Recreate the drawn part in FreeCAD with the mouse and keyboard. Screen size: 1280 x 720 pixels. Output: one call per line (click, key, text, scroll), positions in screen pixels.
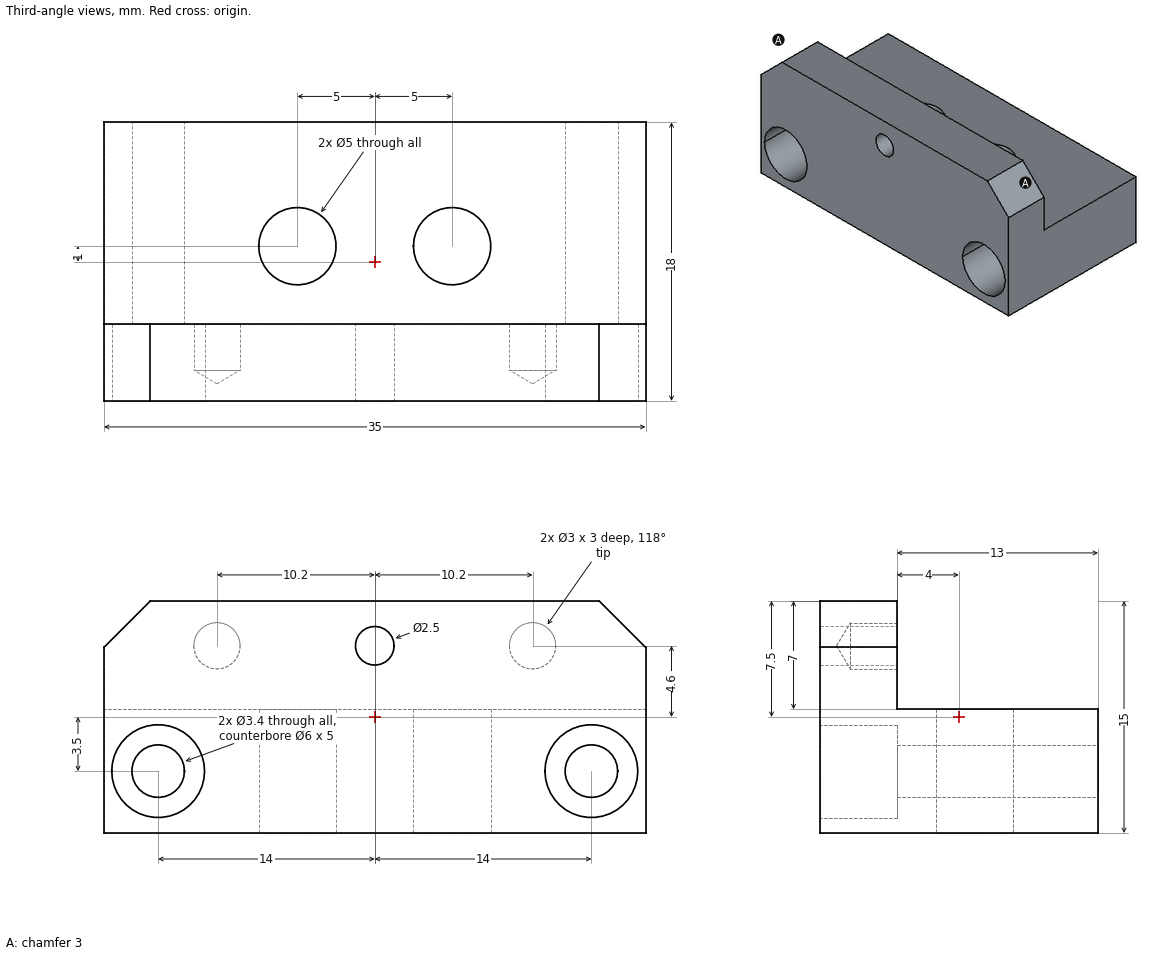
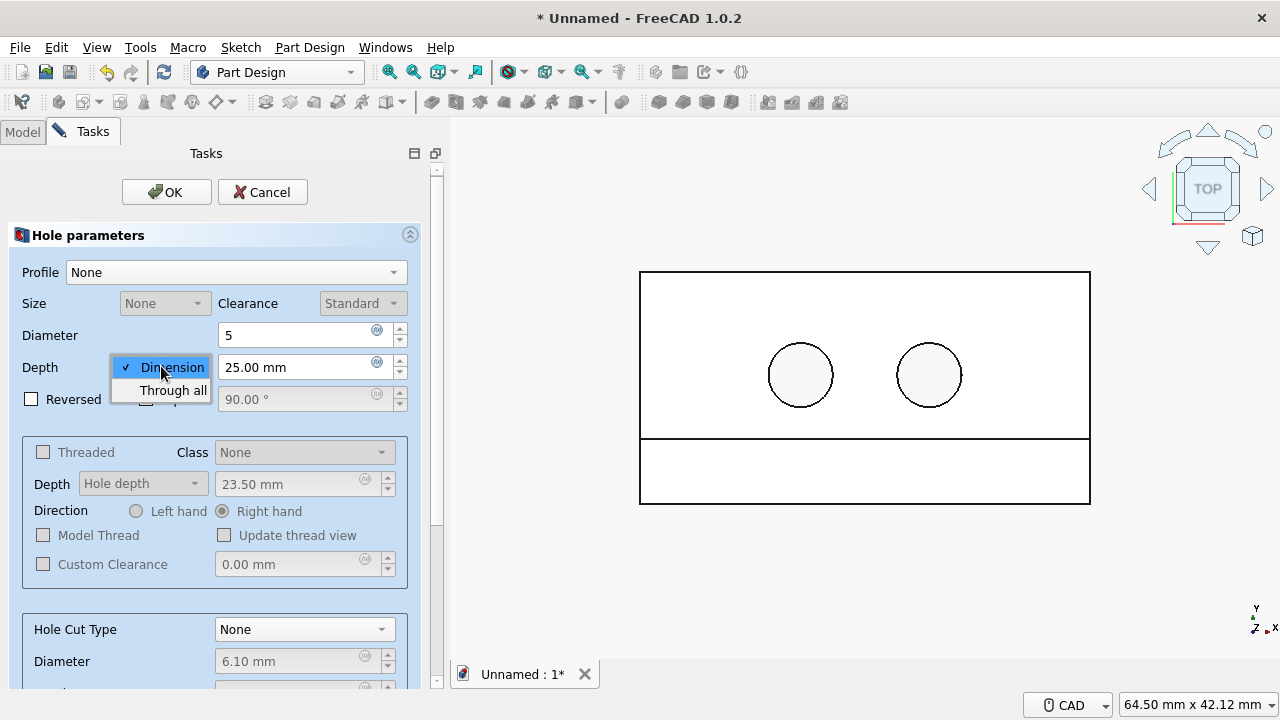
click(160, 390)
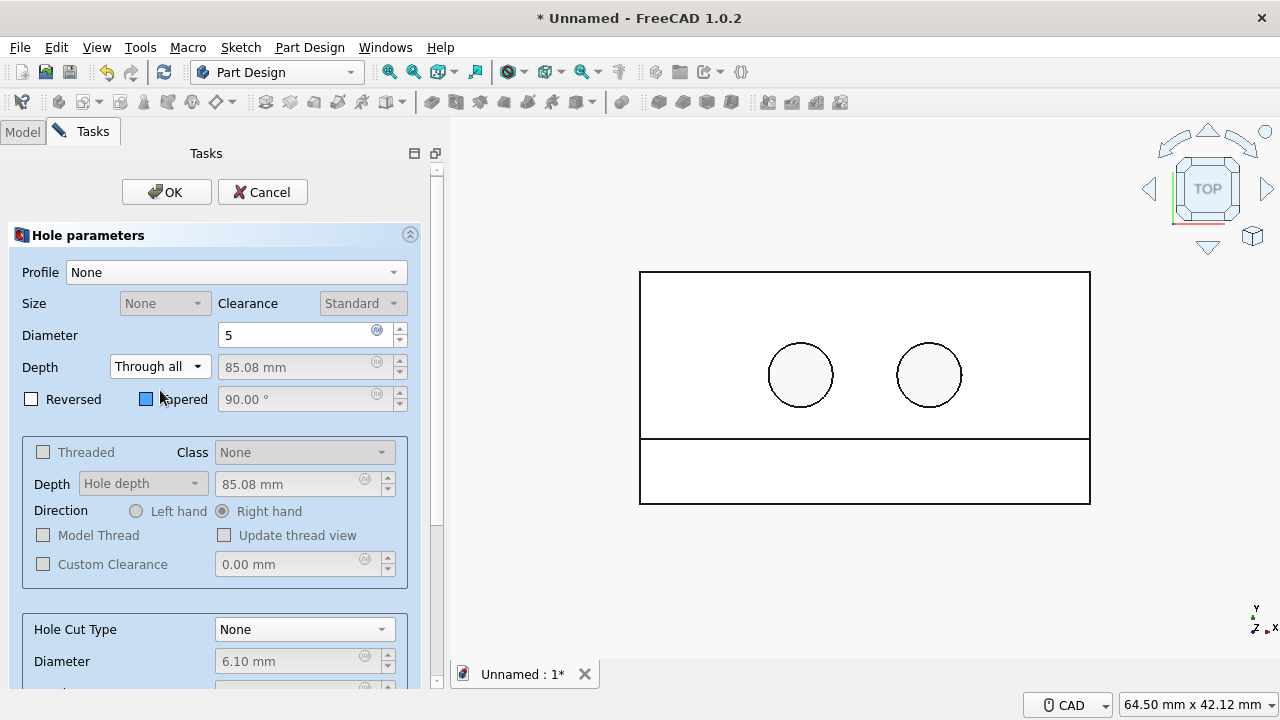
click(167, 192)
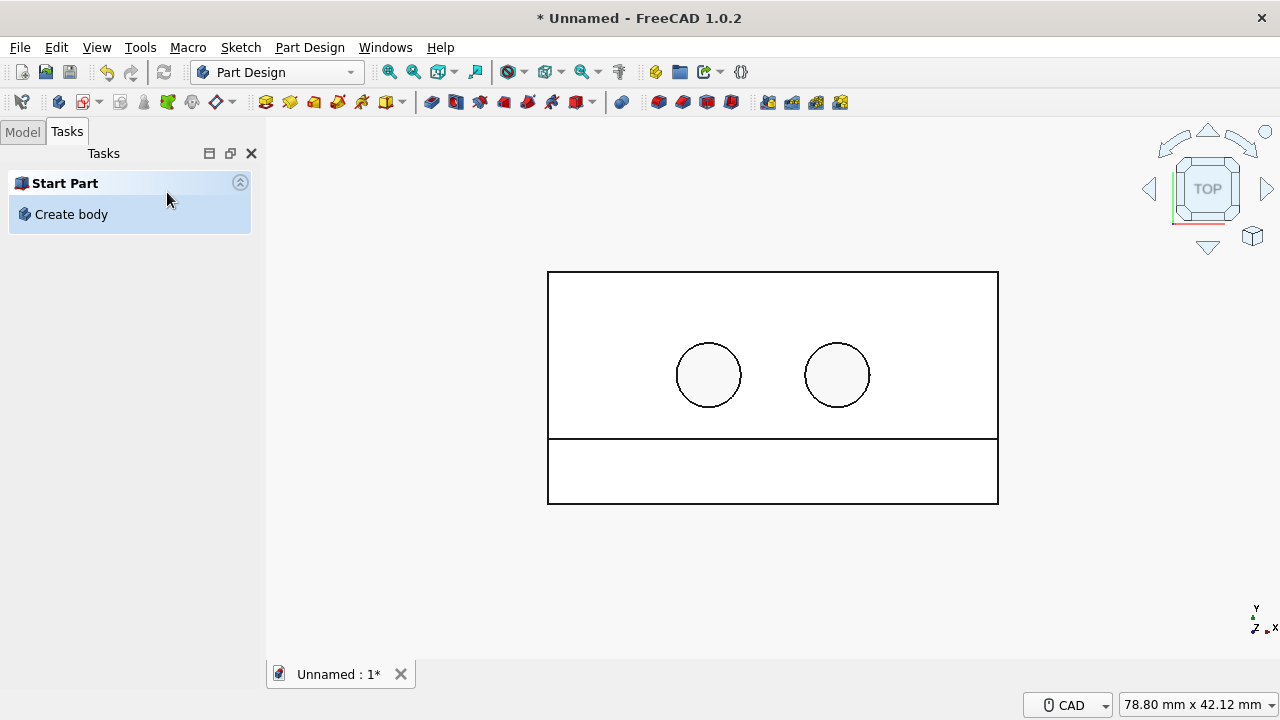
click(390, 72)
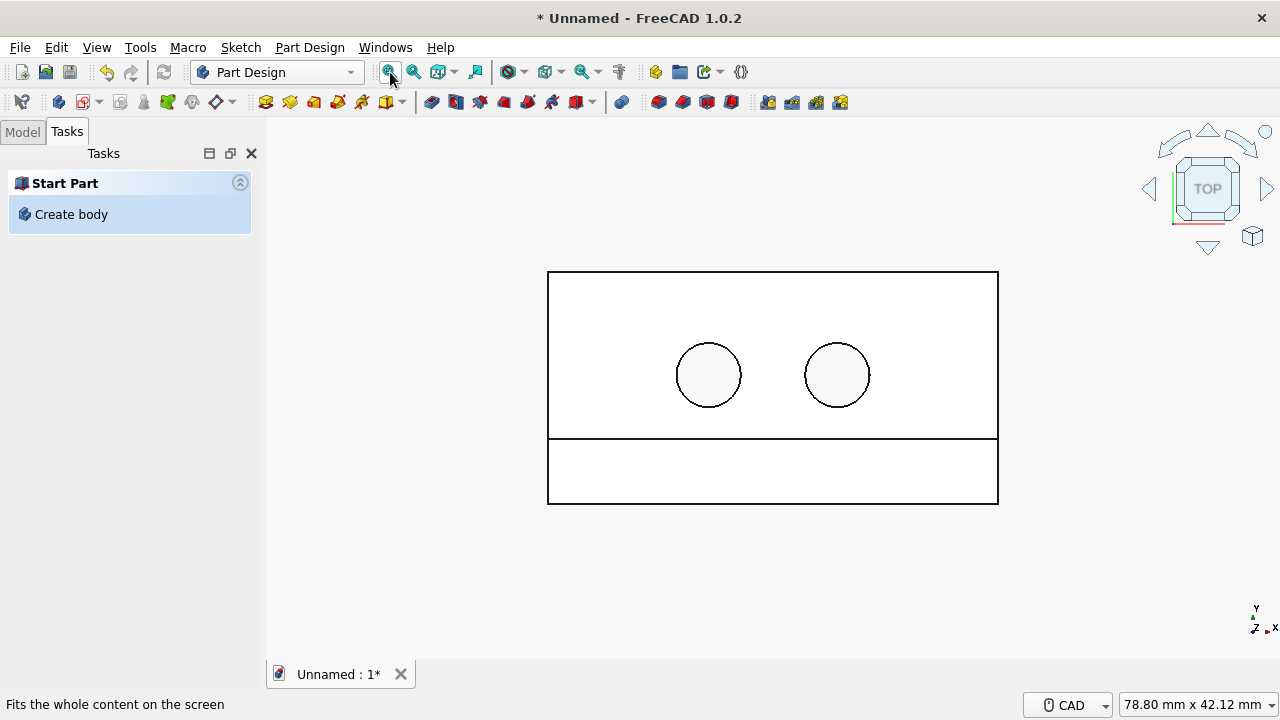
key(4)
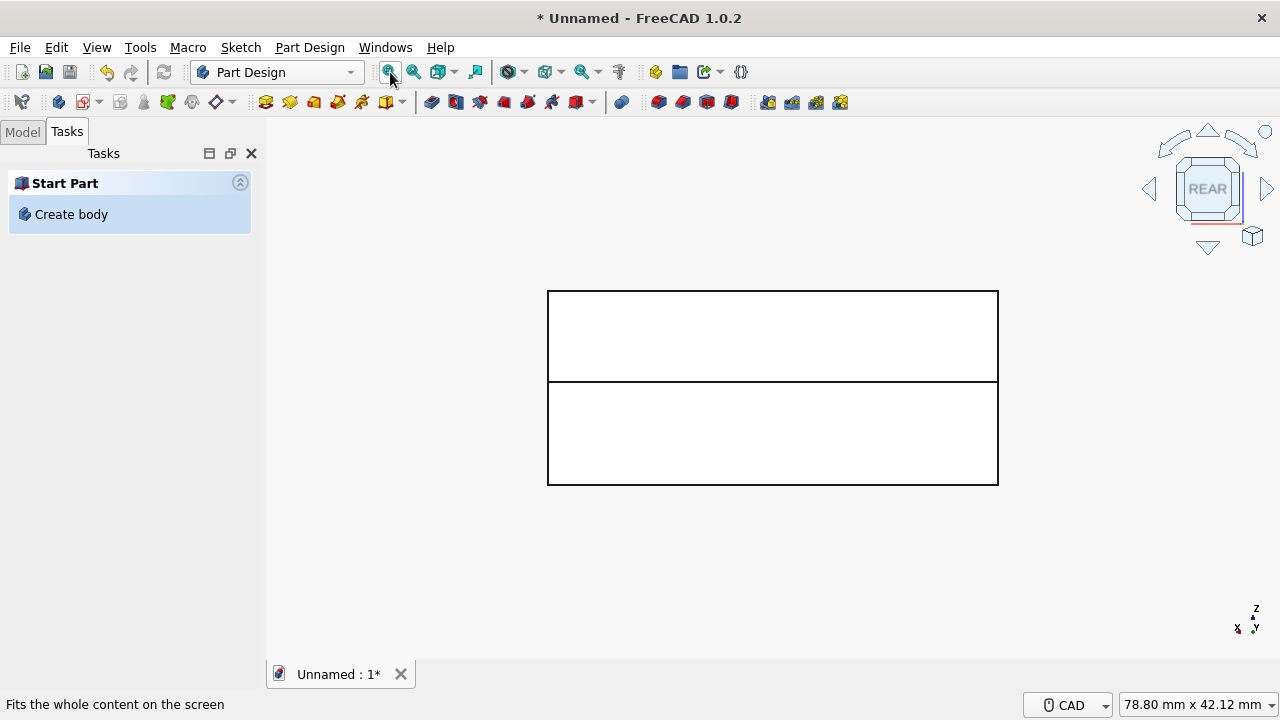
key(v)
key(f)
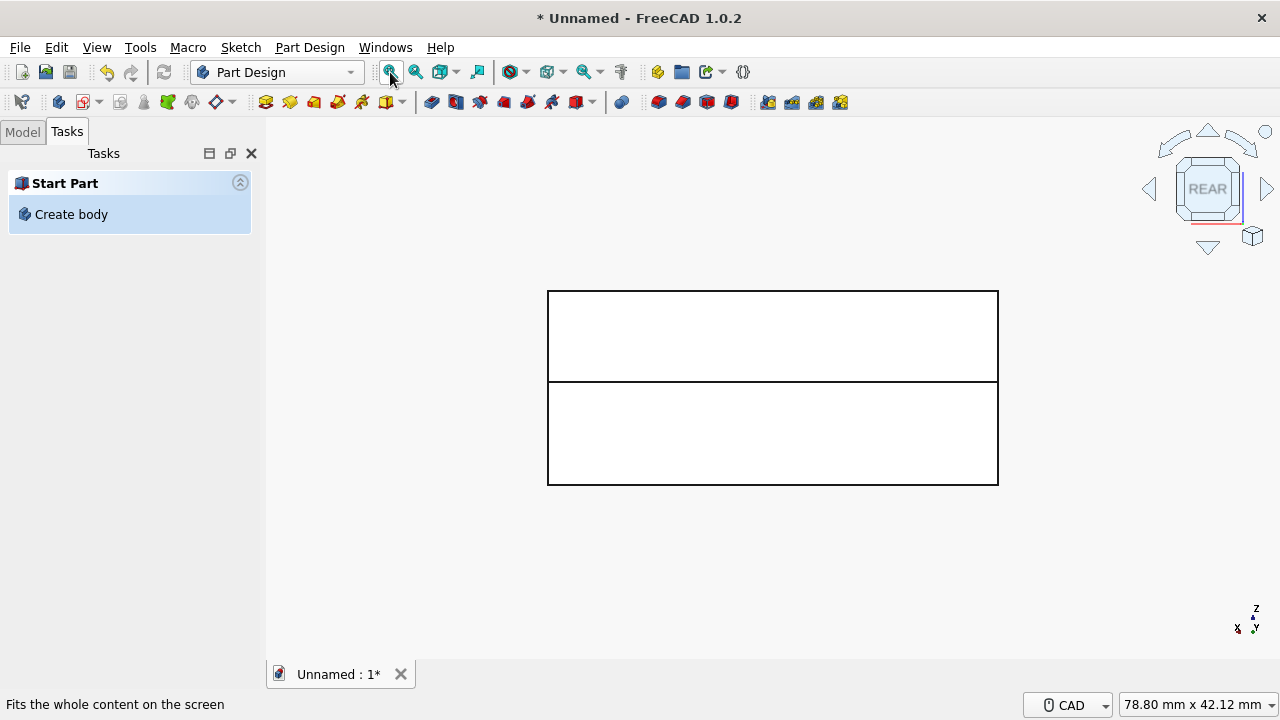
click(644, 336)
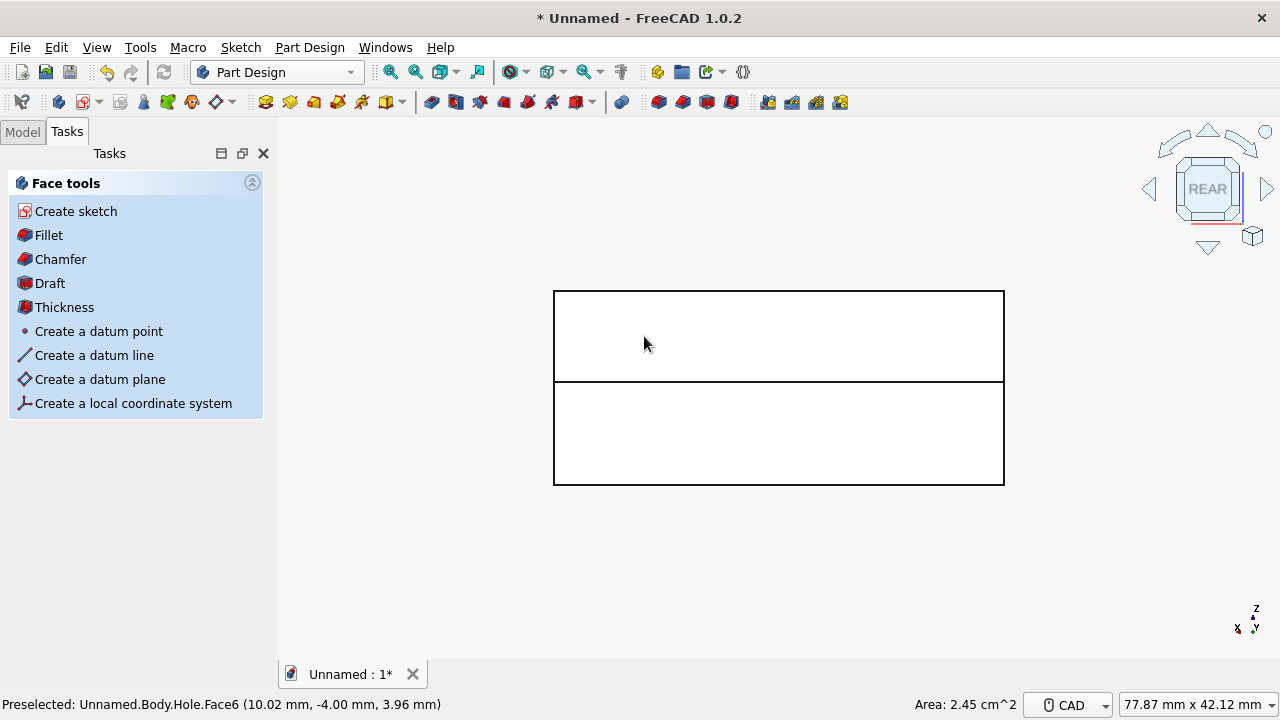
click(84, 102)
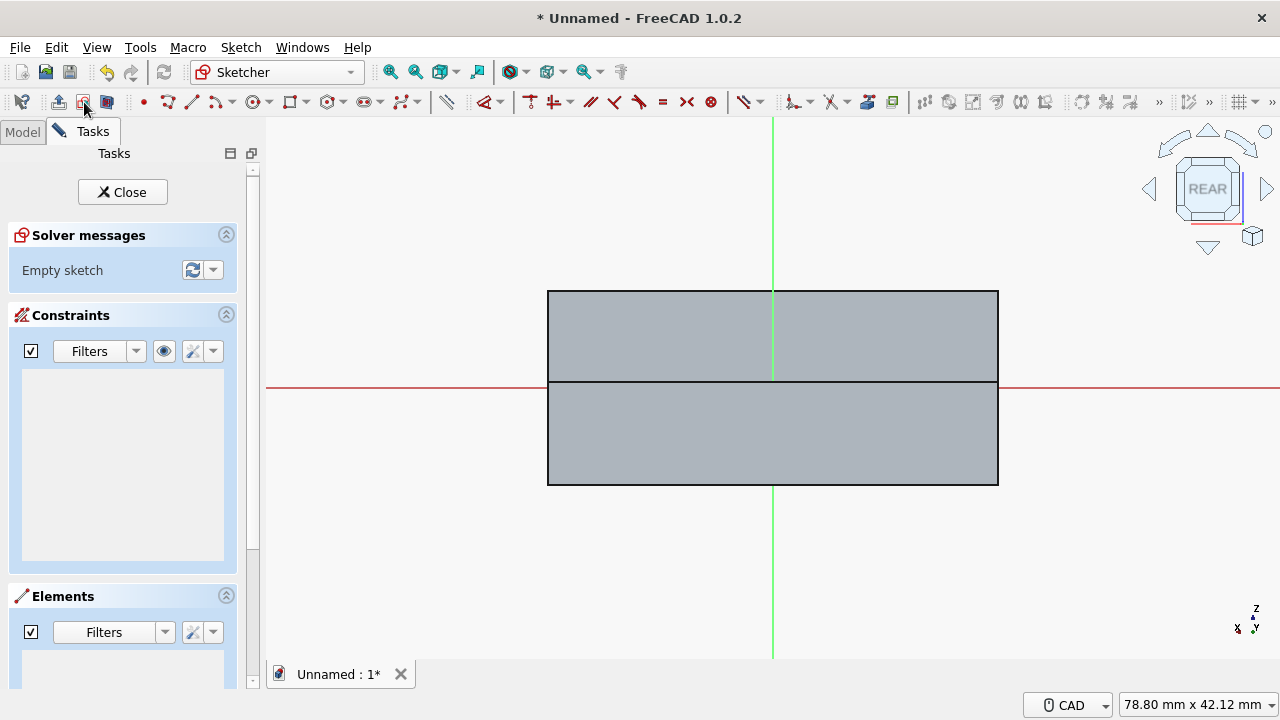
scroll(856, 301, up, 3)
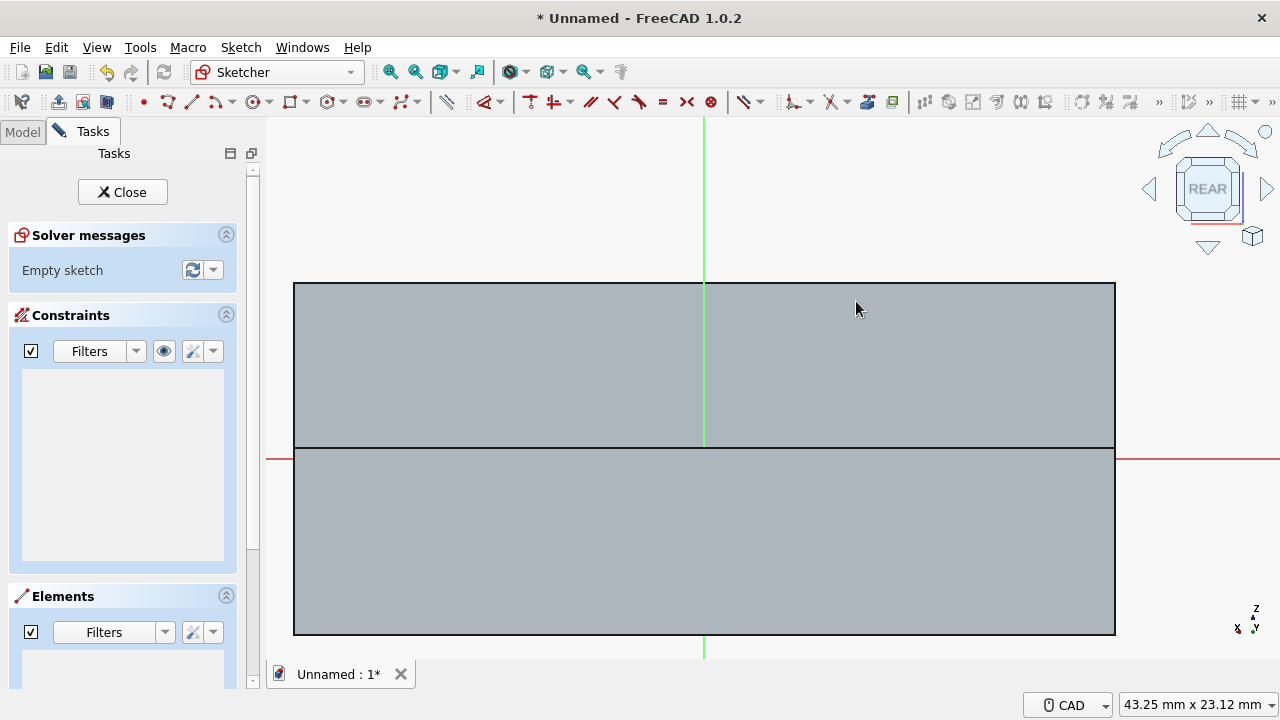
key(g)
key(c)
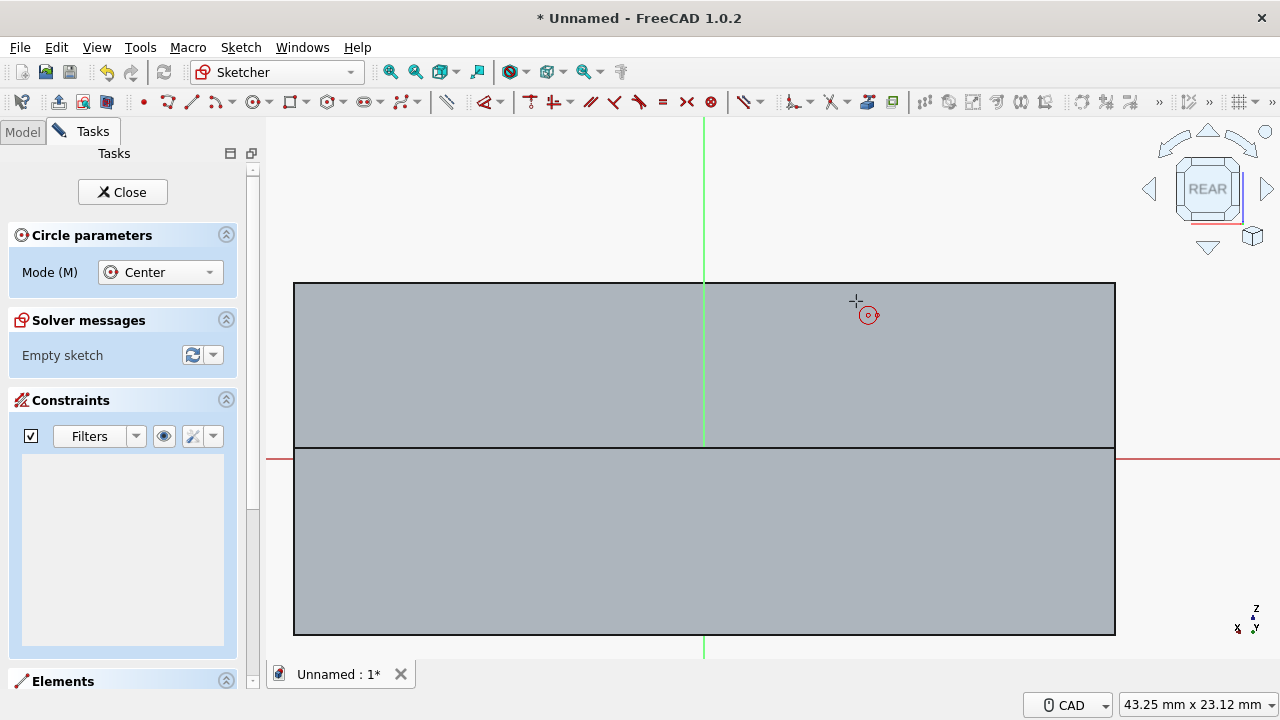
click(465, 351)
click(490, 327)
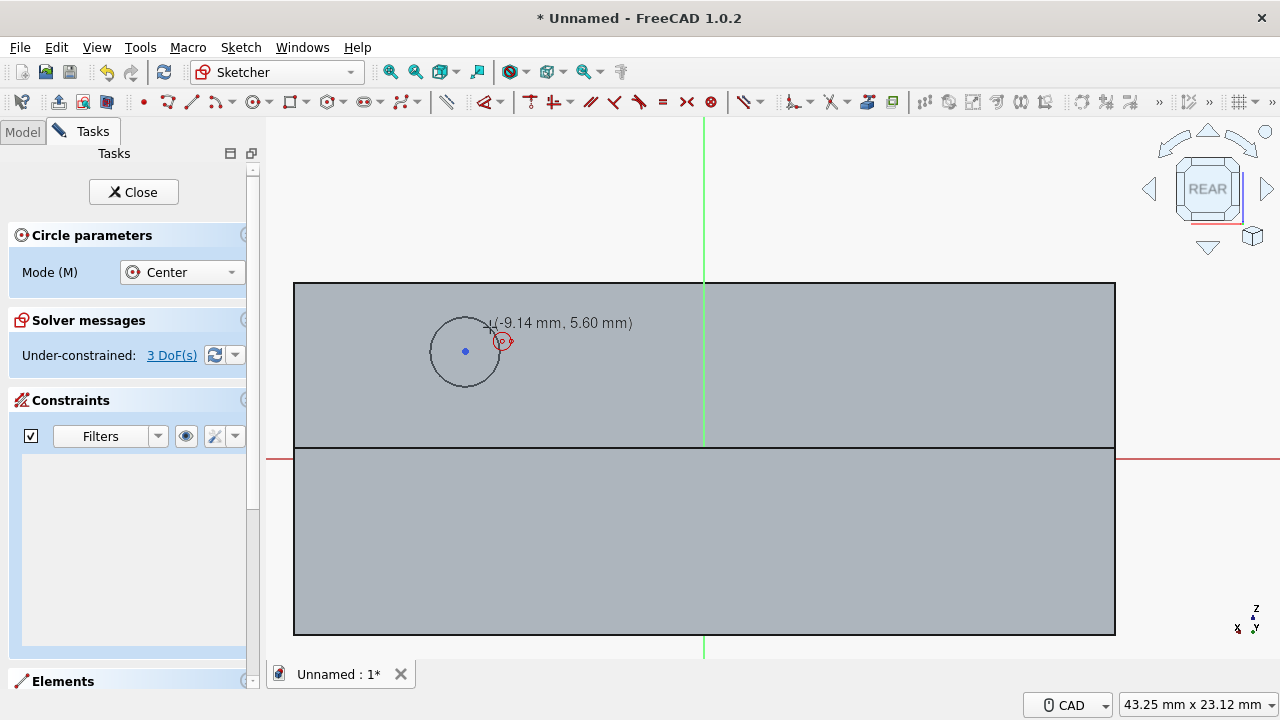
click(943, 351)
click(968, 327)
key(Escape)